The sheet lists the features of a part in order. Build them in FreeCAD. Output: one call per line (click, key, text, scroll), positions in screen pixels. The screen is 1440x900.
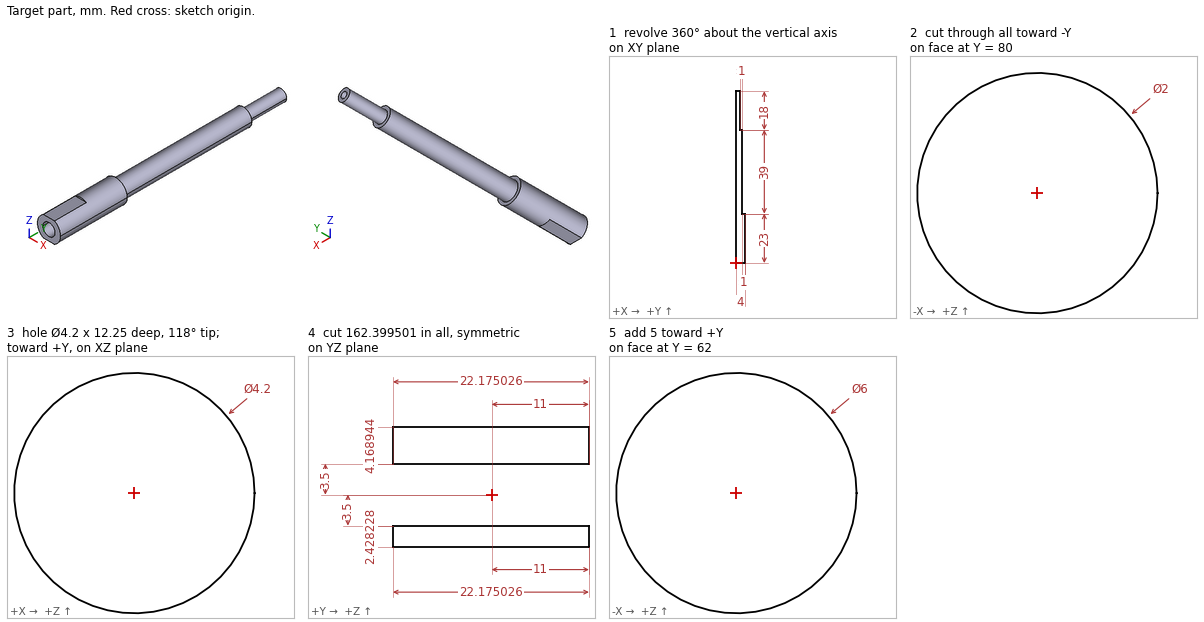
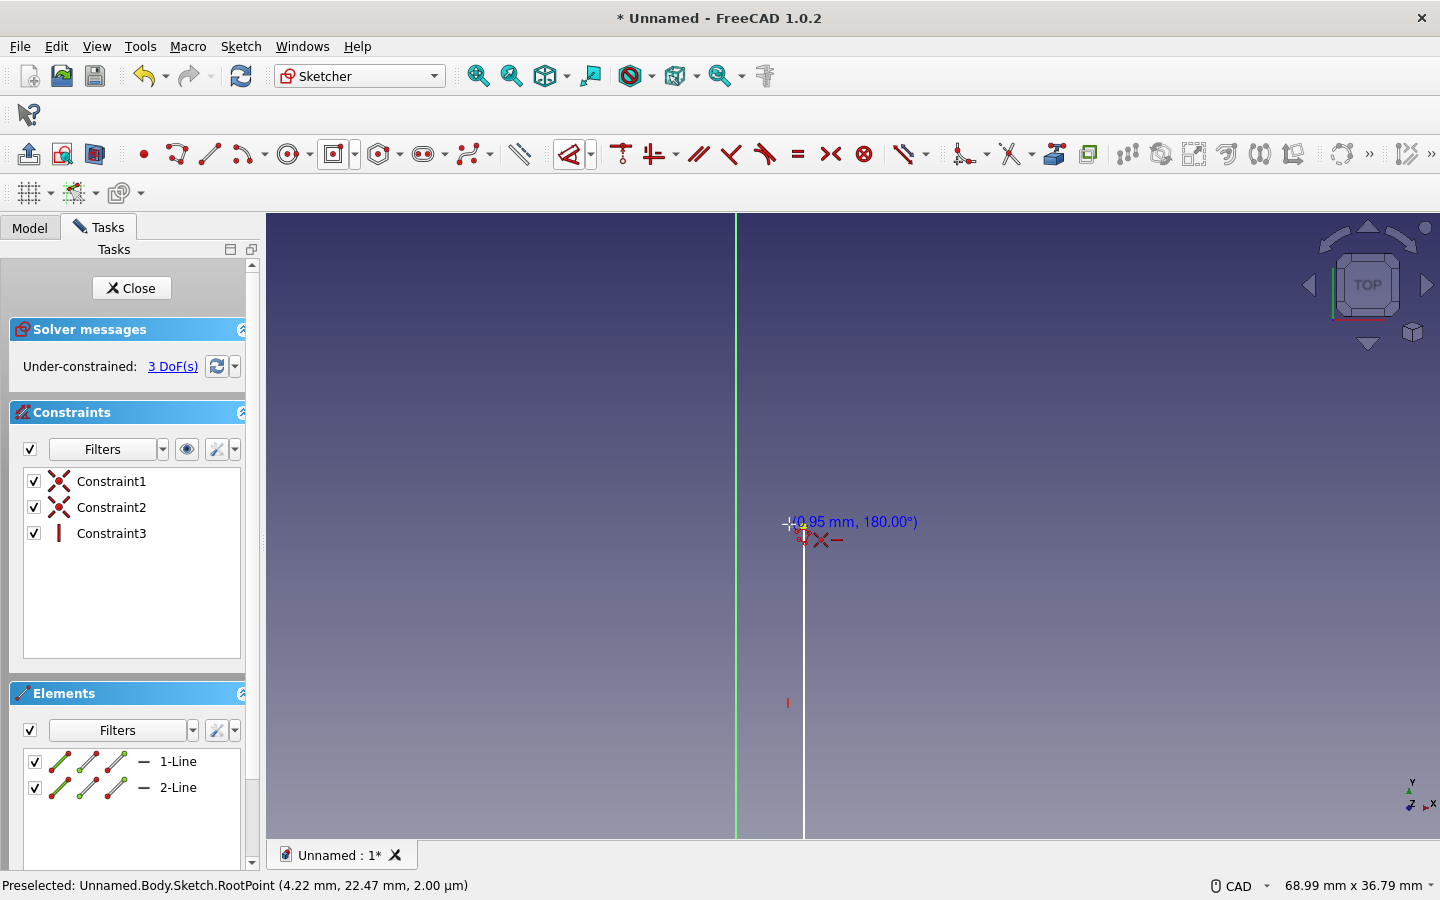
click(787, 522)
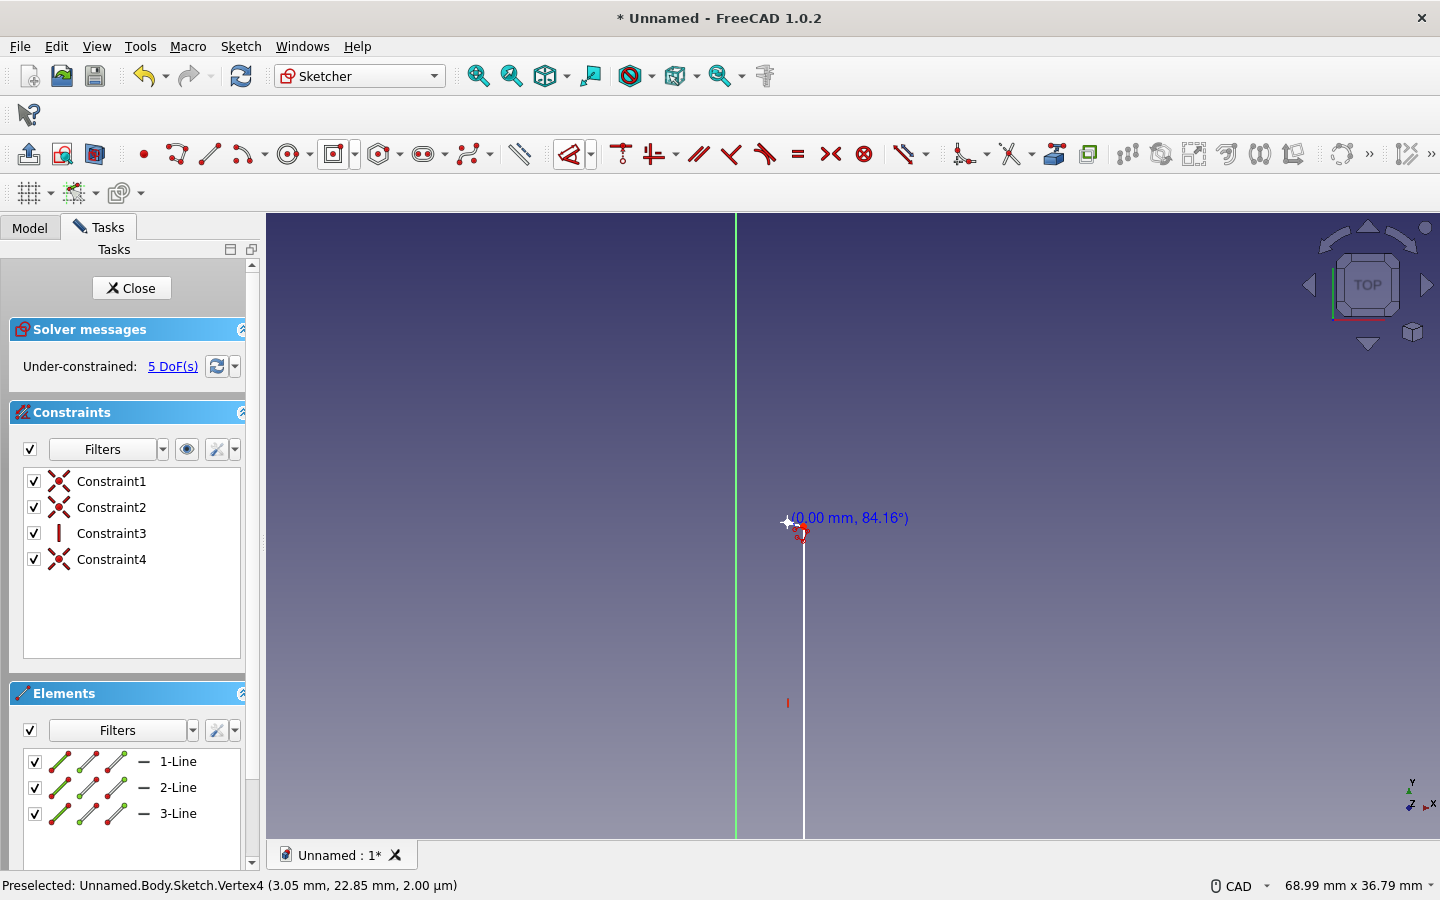
scroll(791, 653, down, 6)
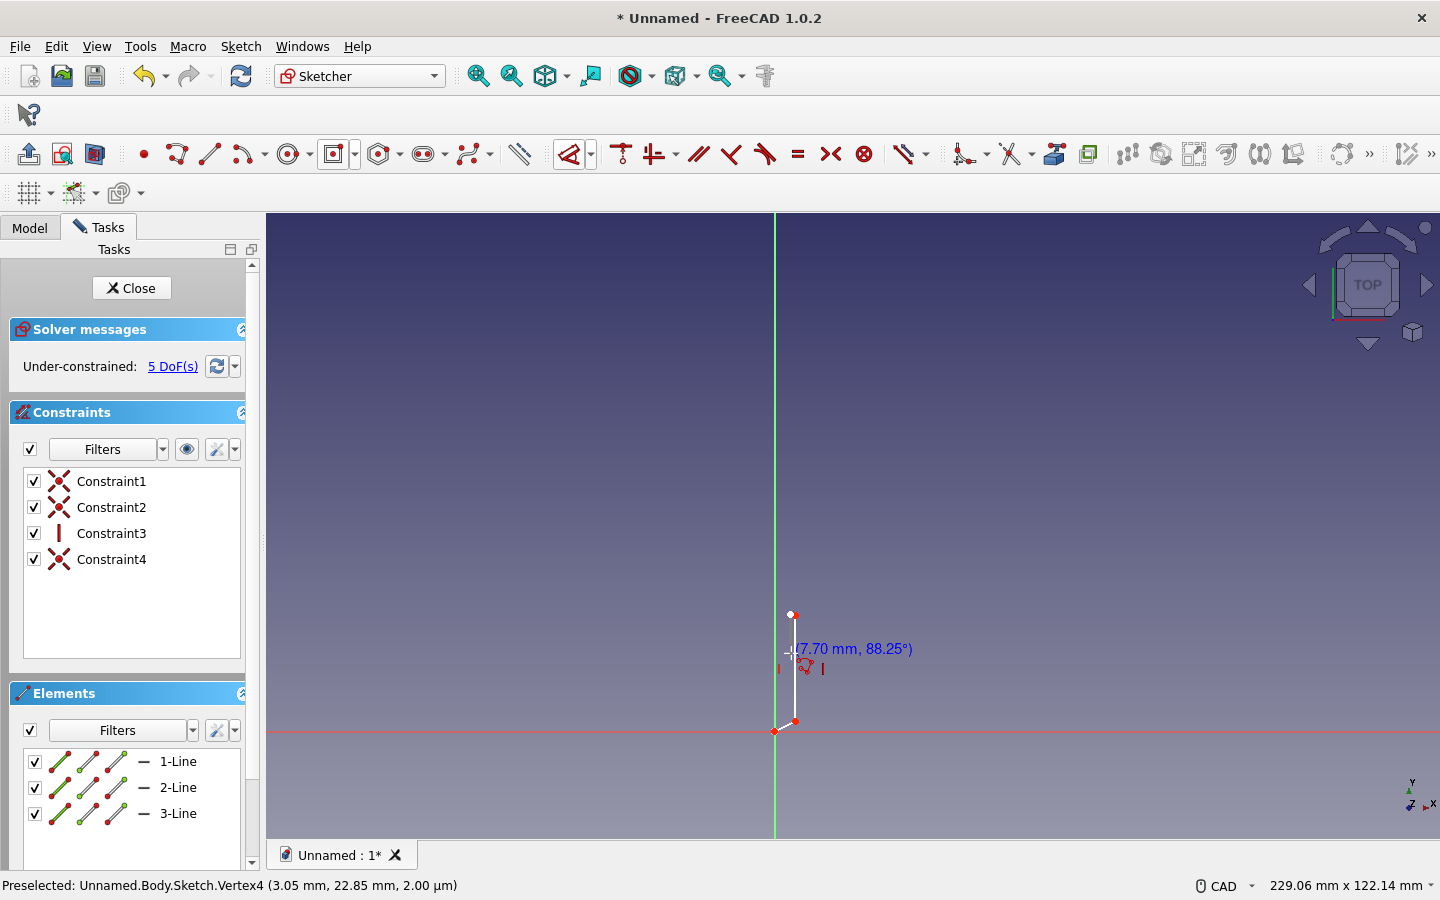
click(790, 414)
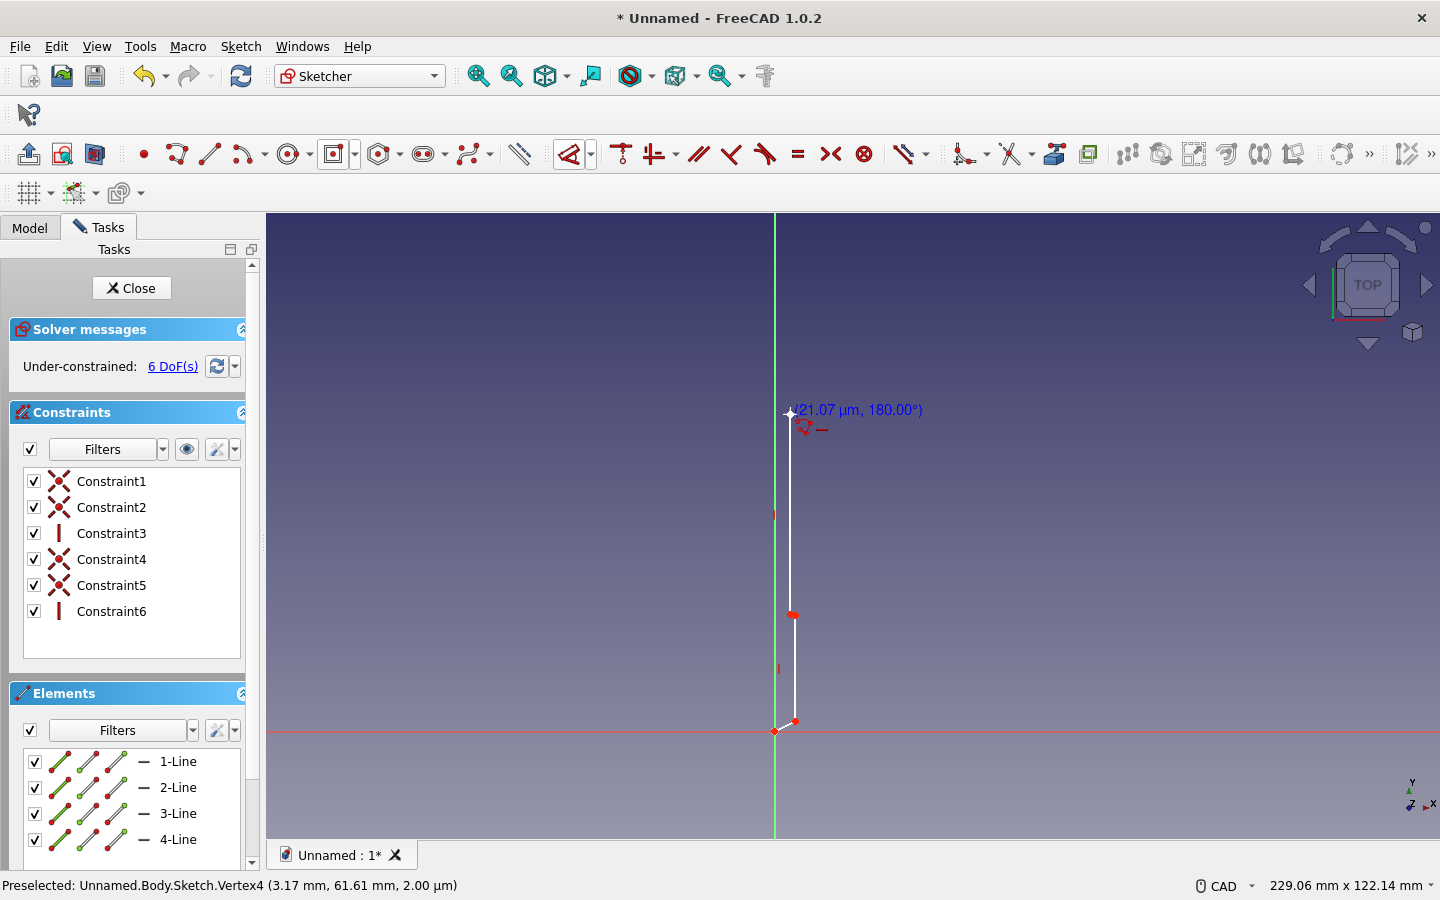
scroll(785, 414, up, 6)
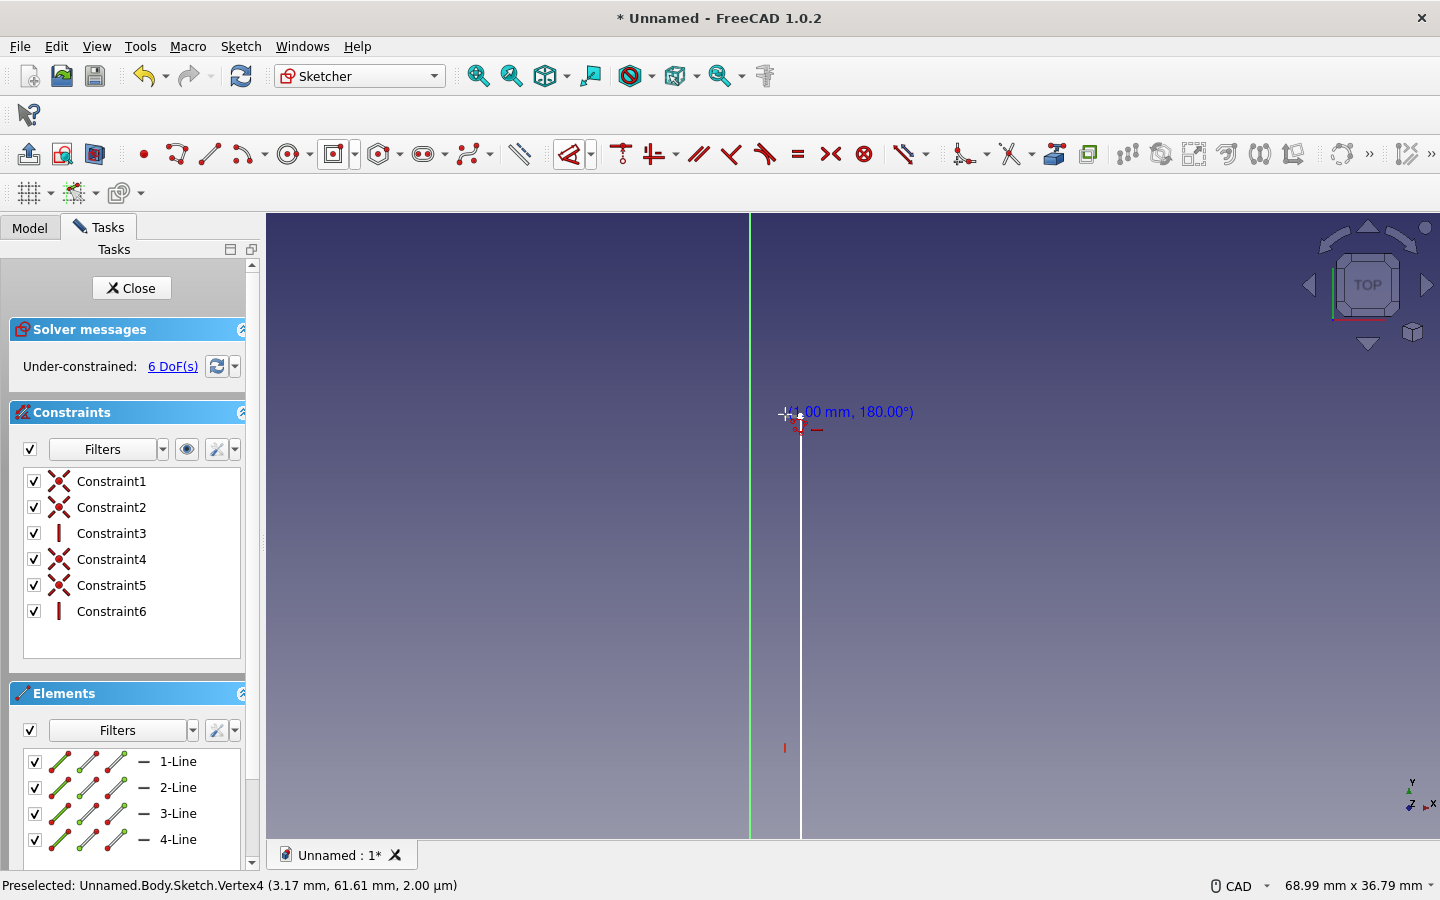
click(784, 413)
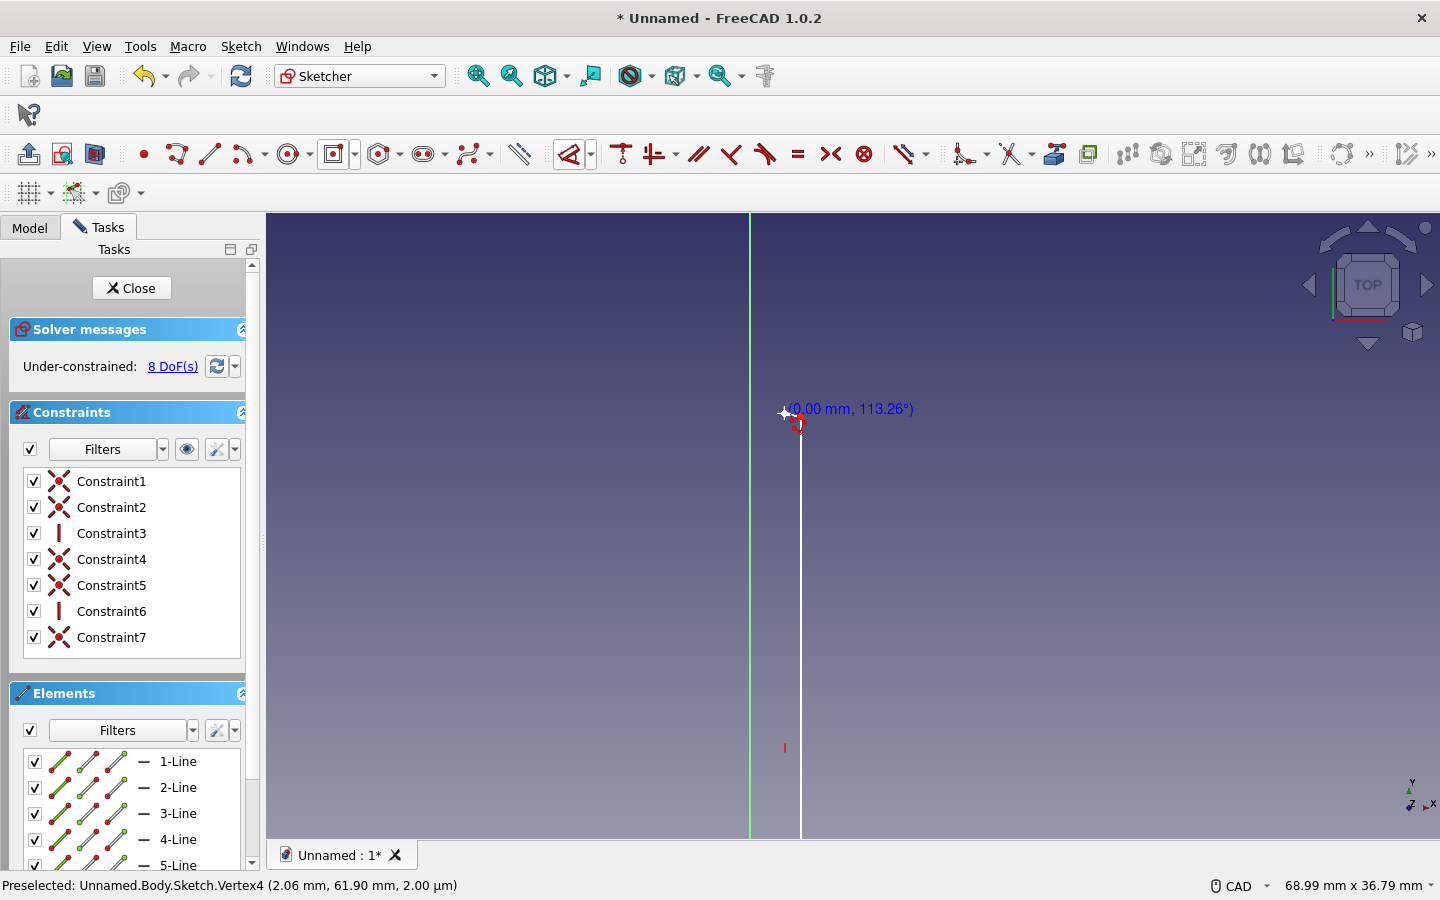
scroll(785, 413, down, 6)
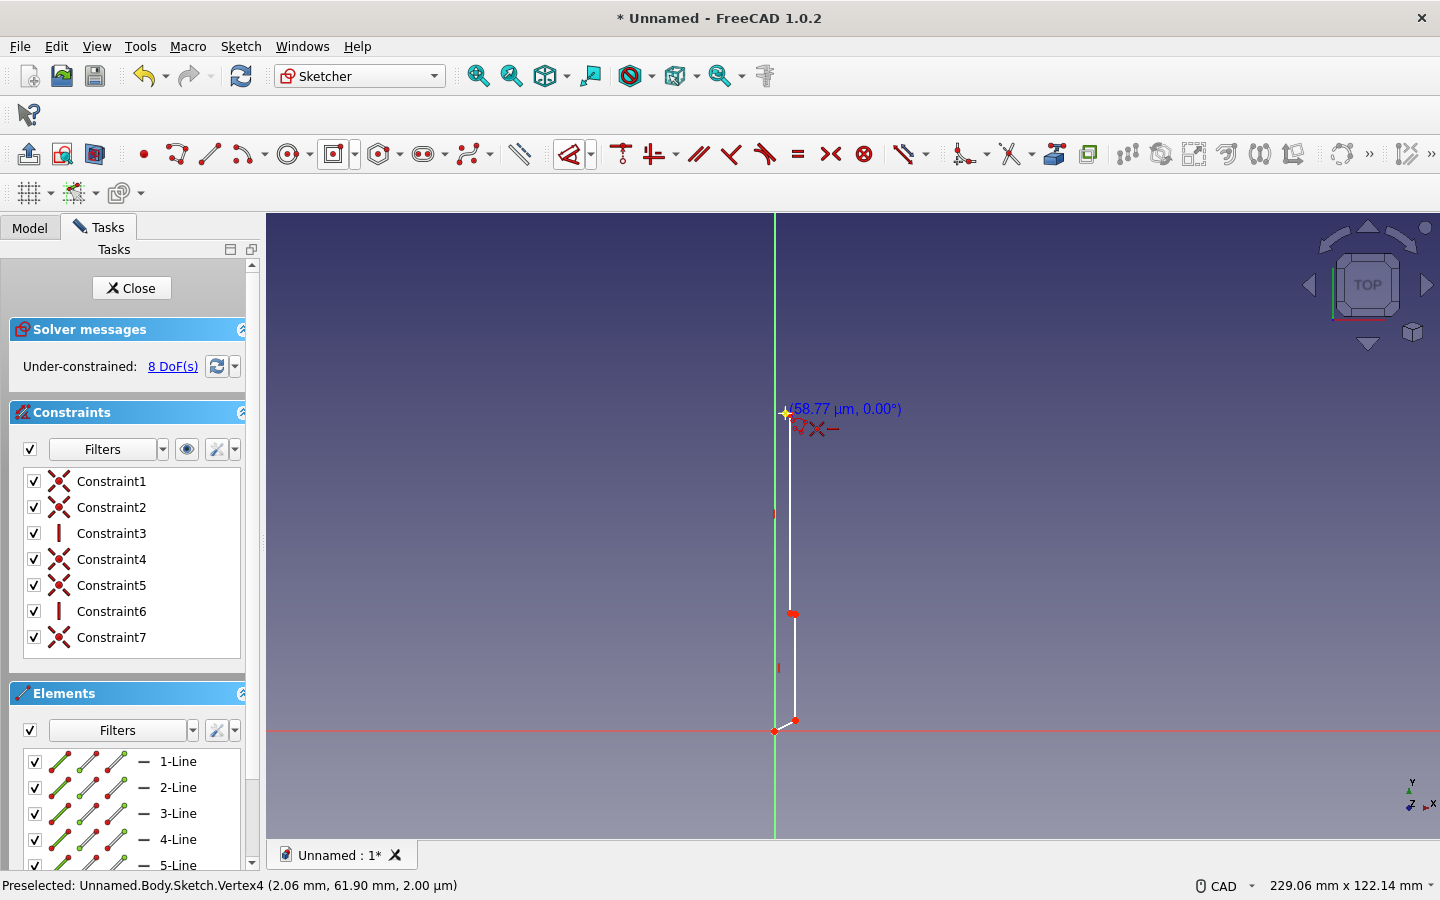
scroll(785, 321, up, 3)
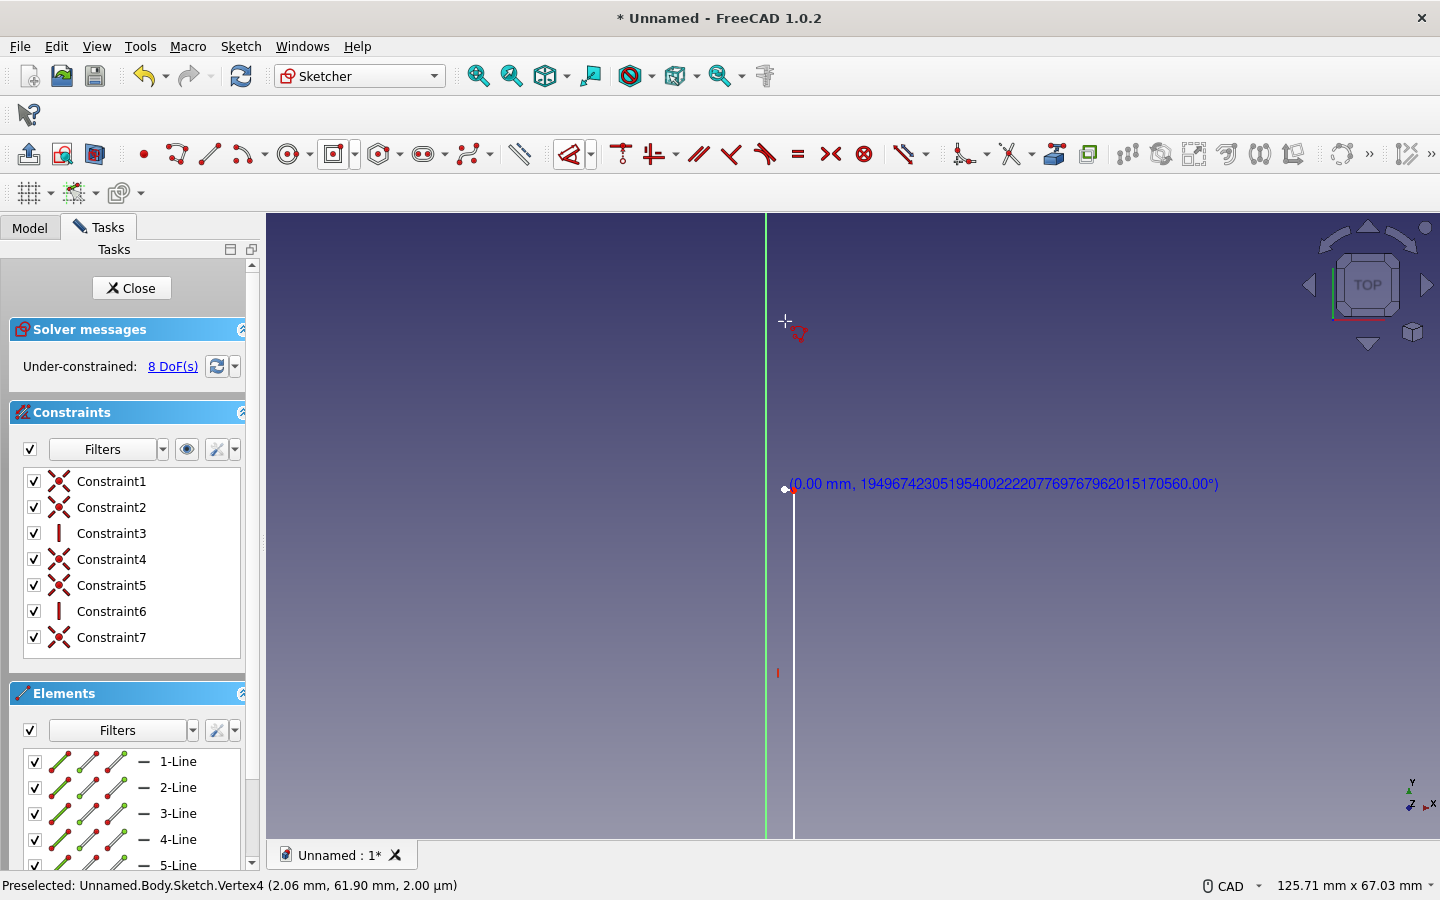
click(785, 321)
click(775, 321)